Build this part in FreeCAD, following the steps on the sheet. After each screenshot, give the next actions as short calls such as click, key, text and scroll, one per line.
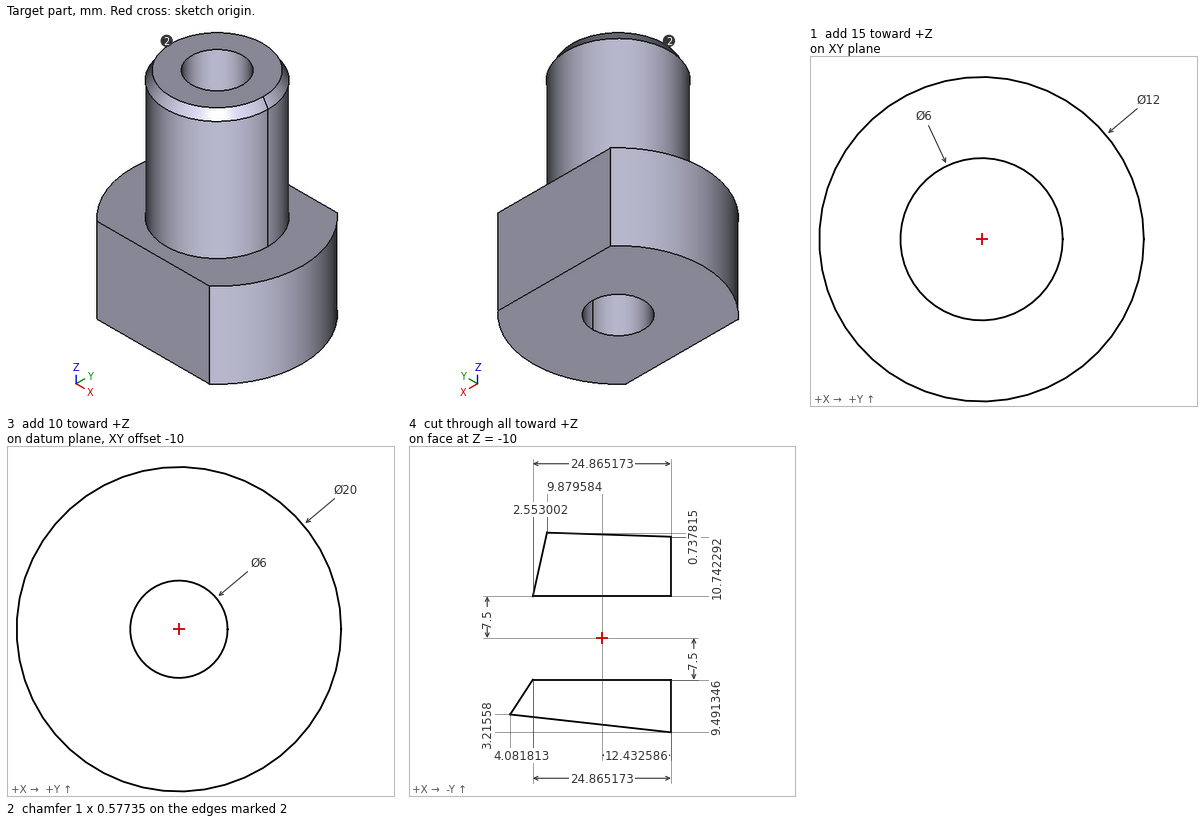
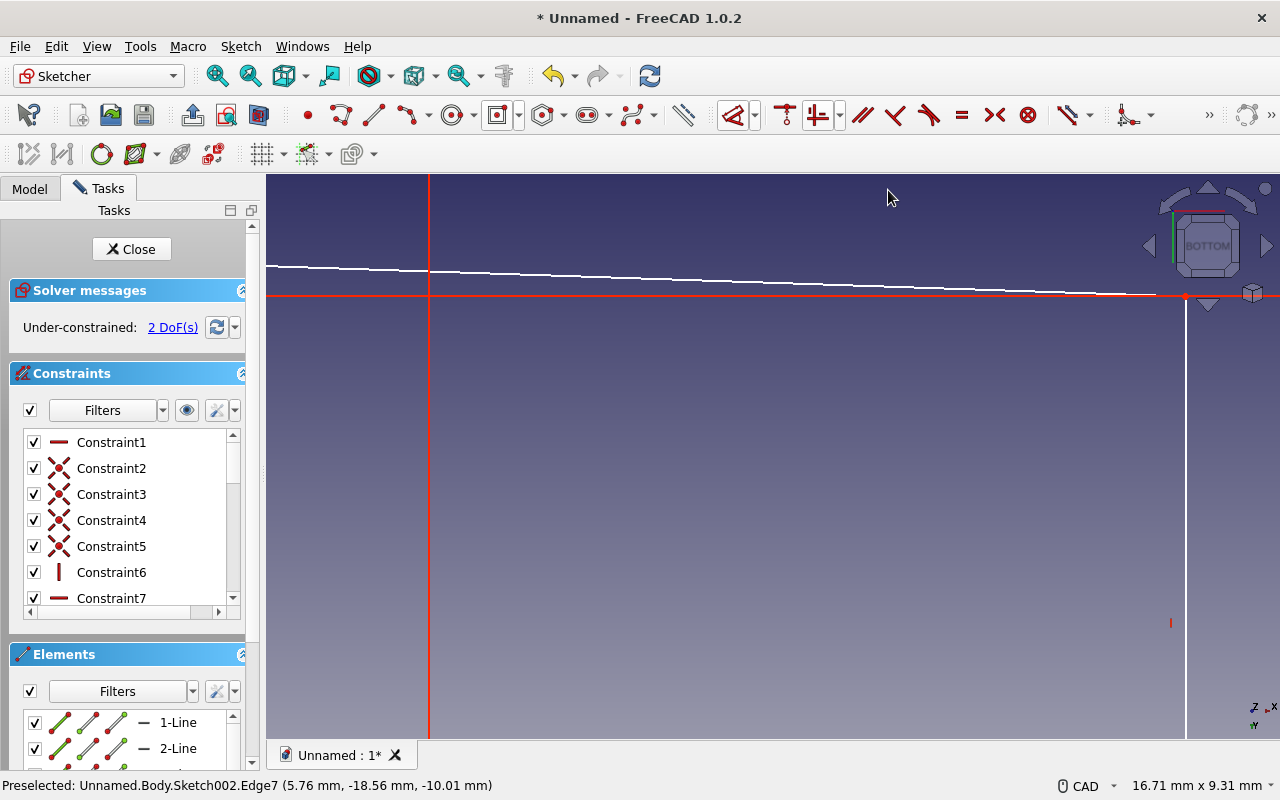
scroll(784, 281, down, 9)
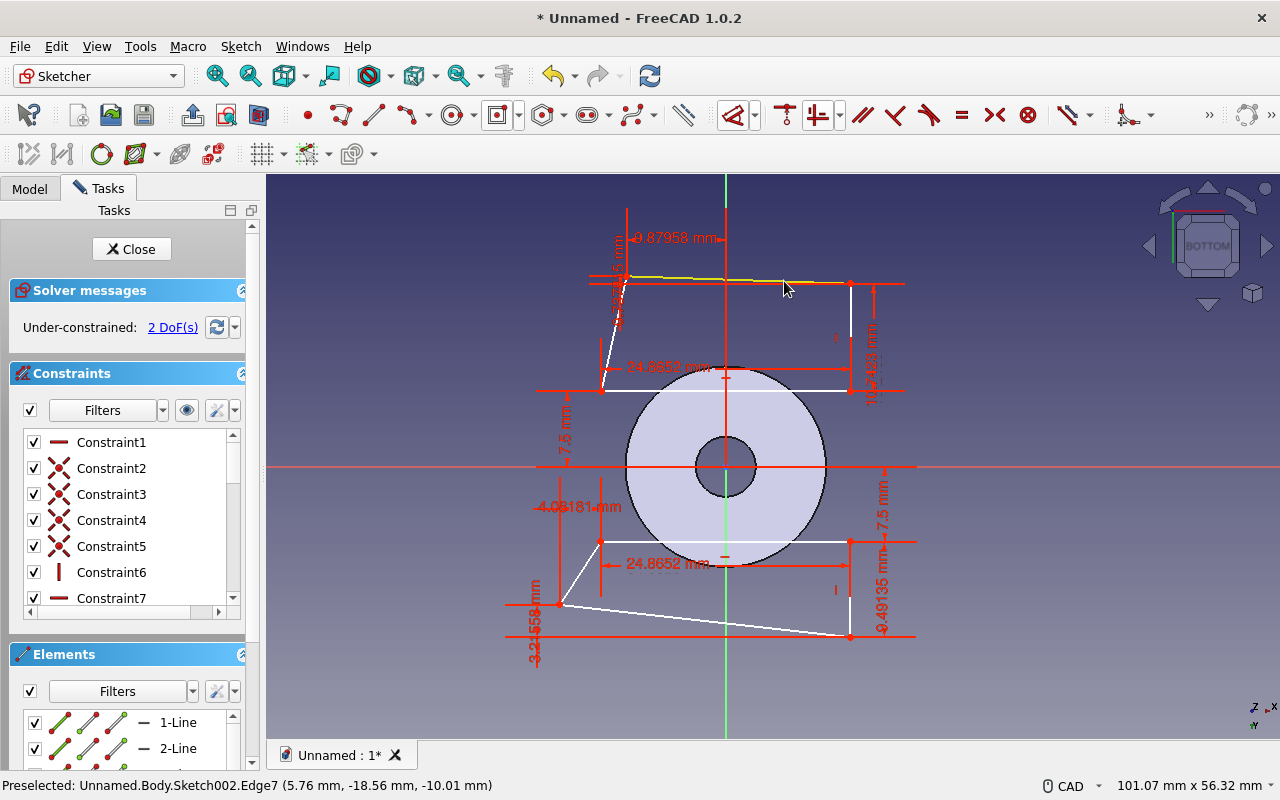
scroll(619, 311, up, 3)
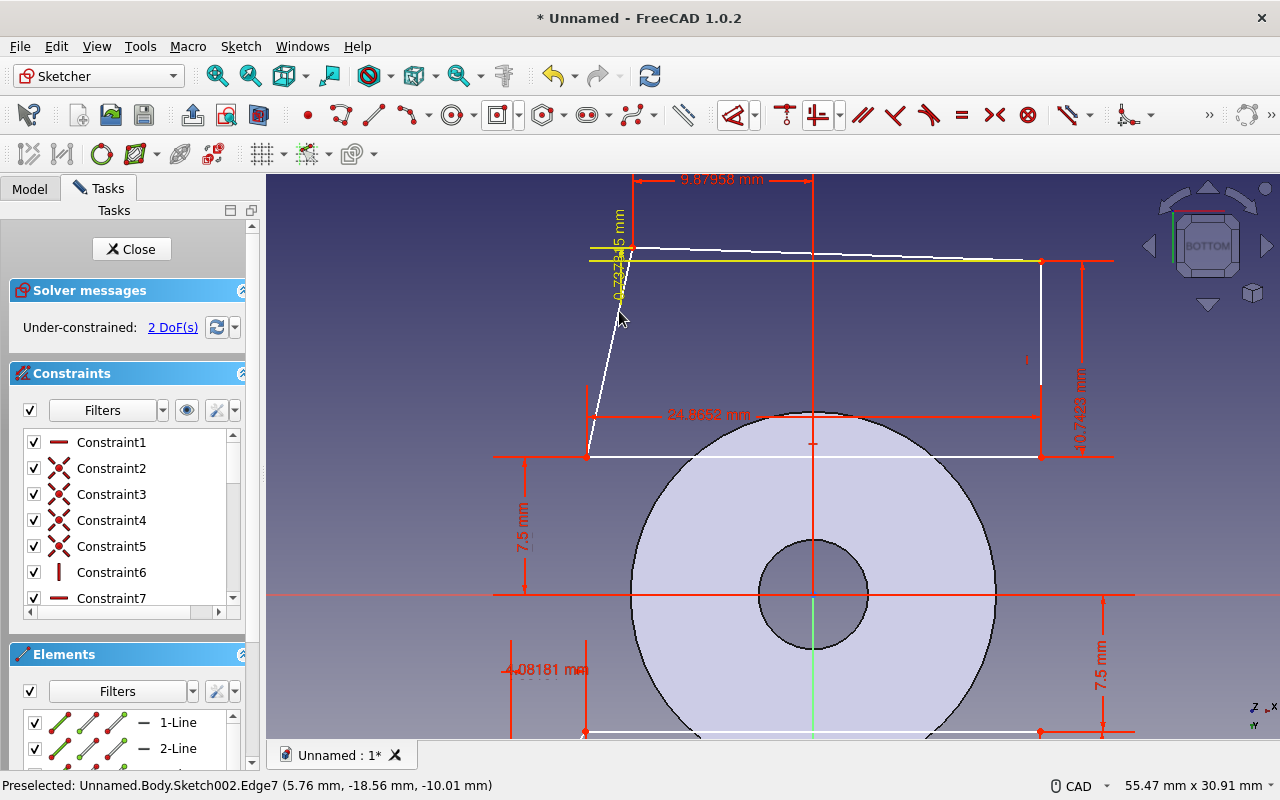
click(619, 311)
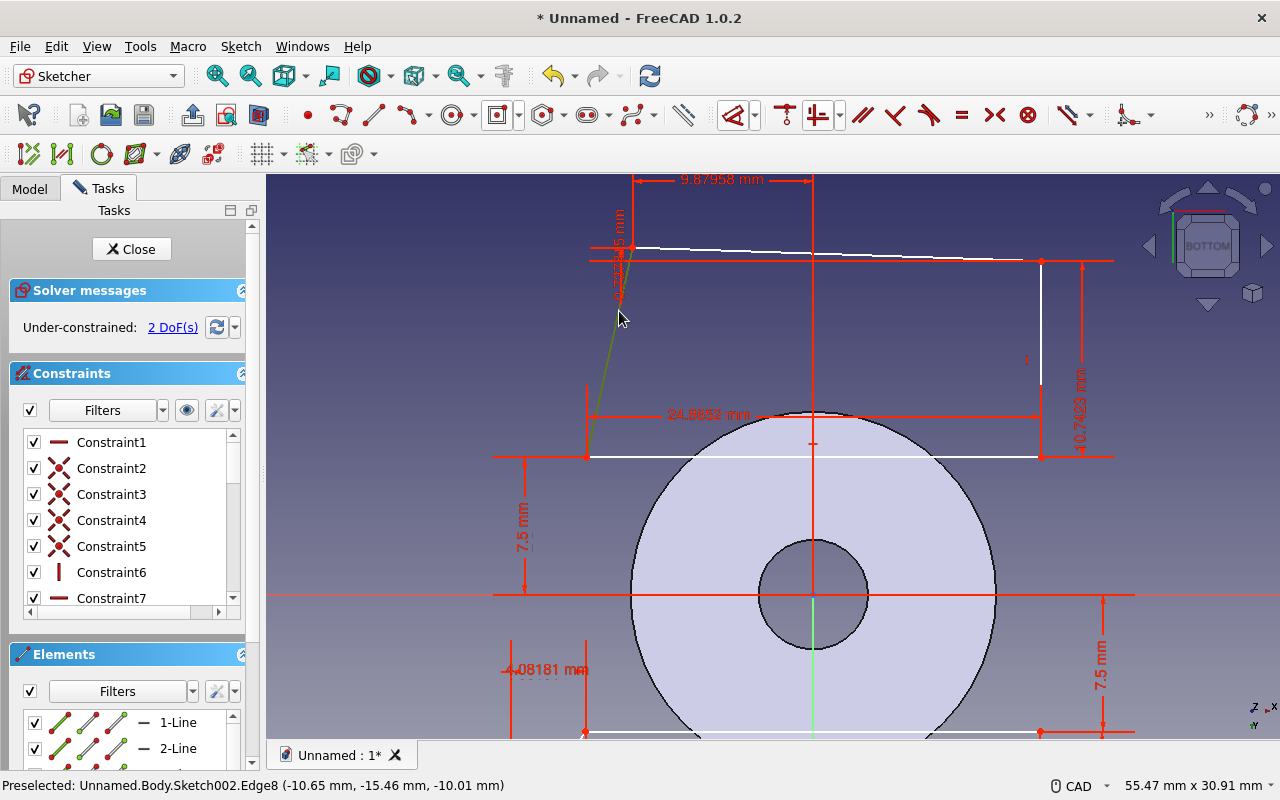
key(l)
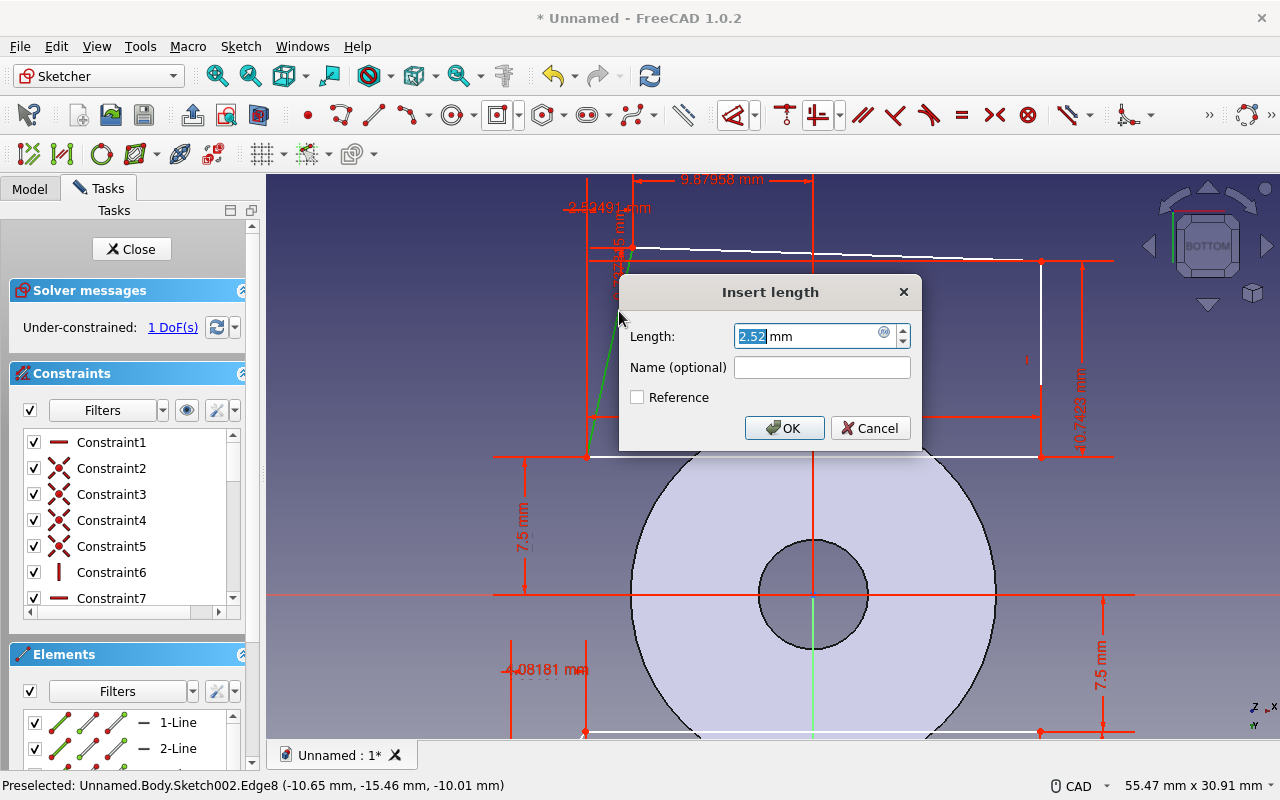
text(2.553002)
key(Return)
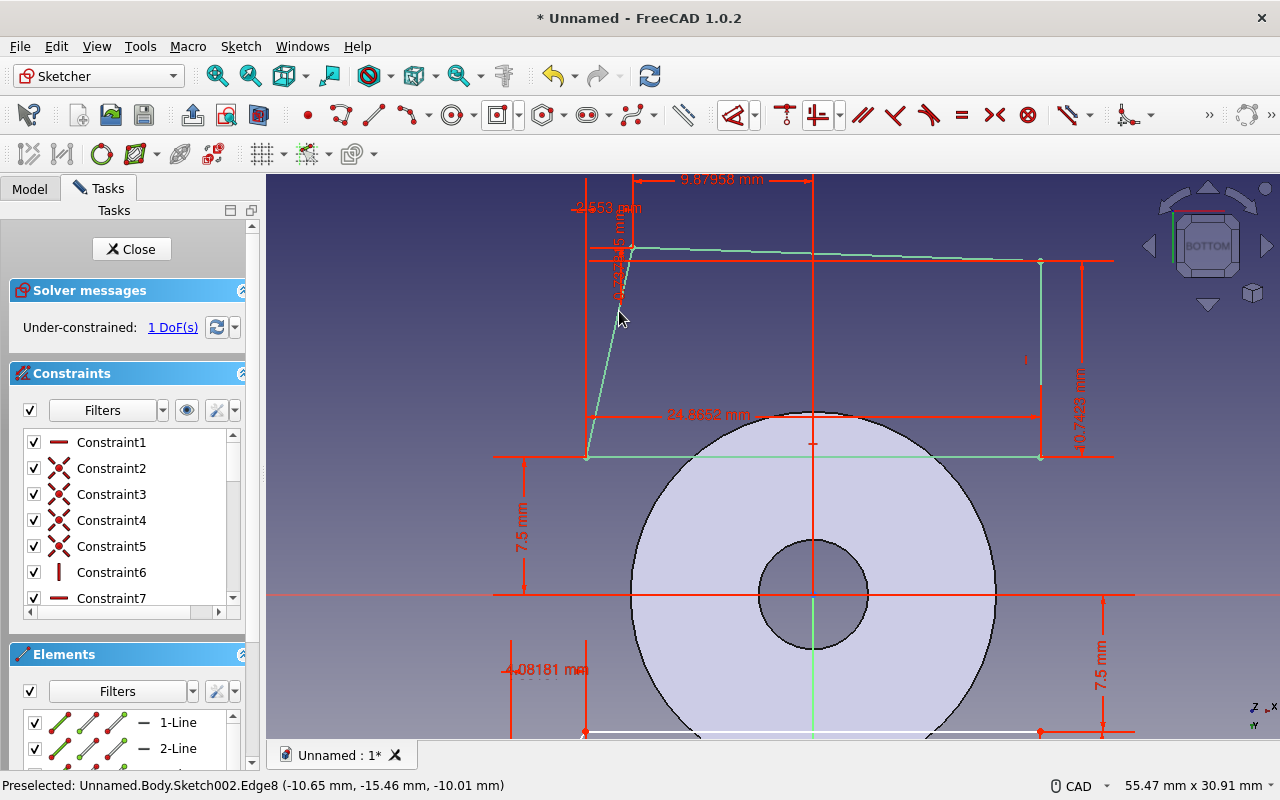
scroll(617, 311, down, 3)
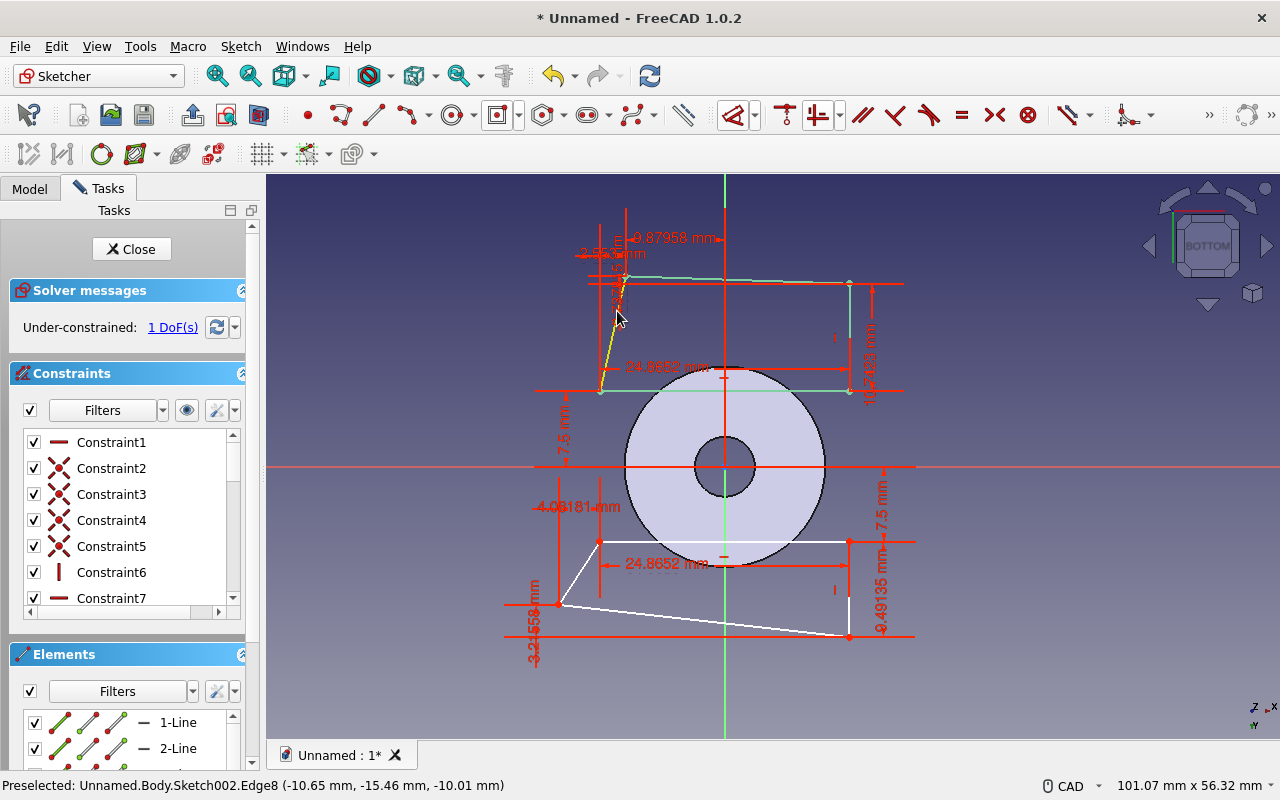
click(849, 542)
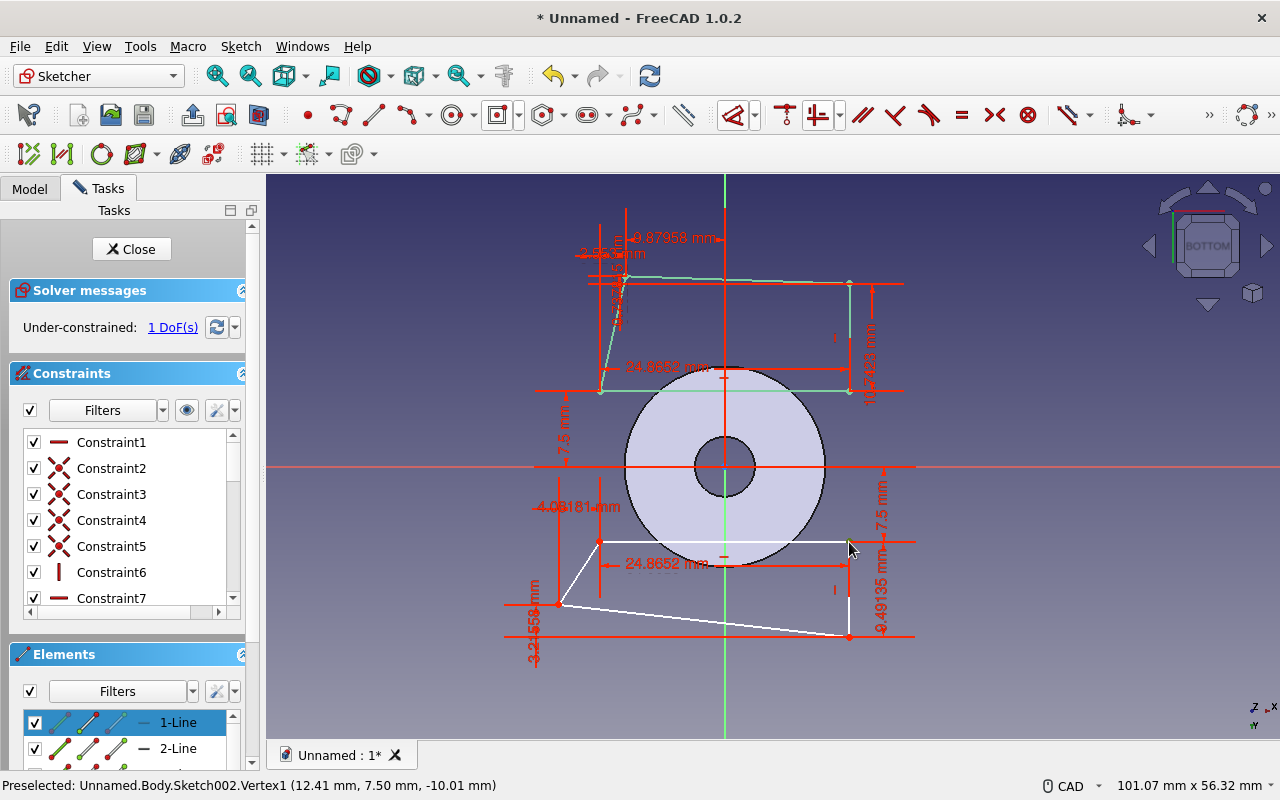
click(754, 116)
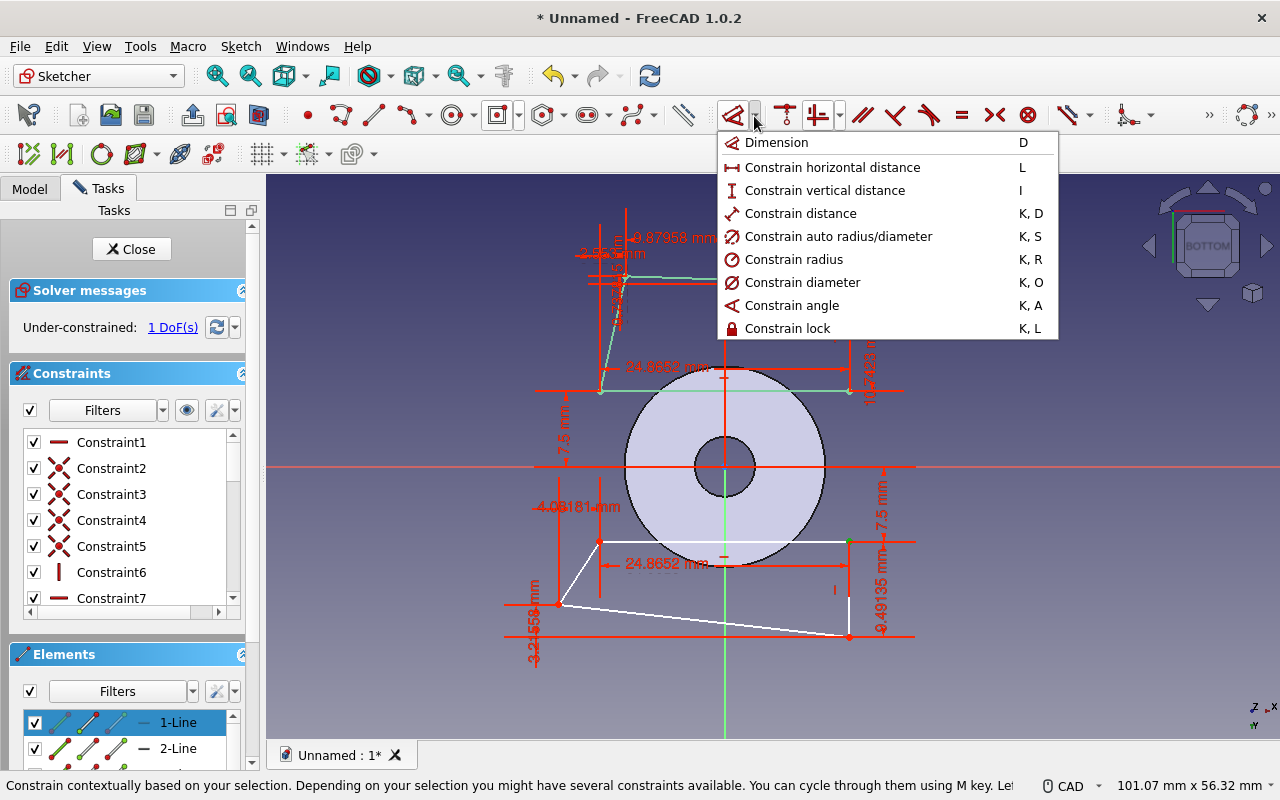
click(888, 168)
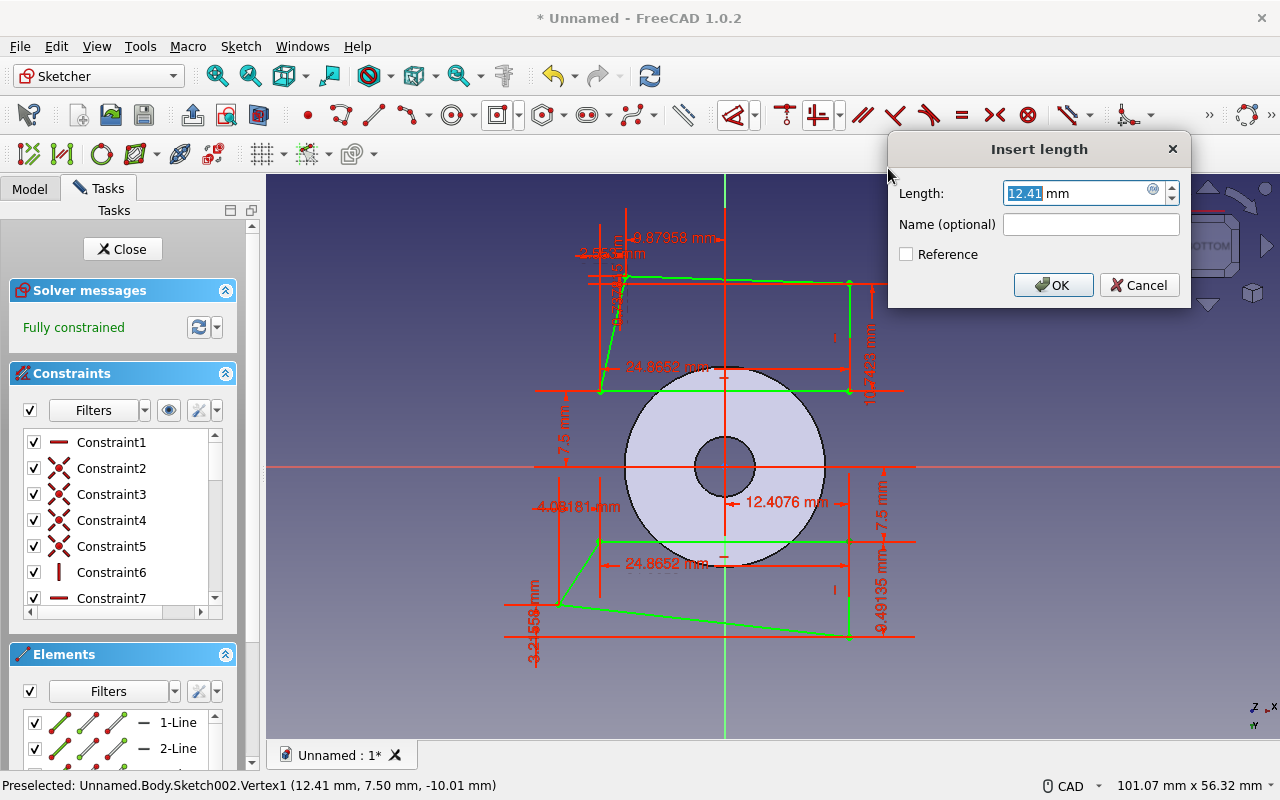
text(12.432586)
key(Return)